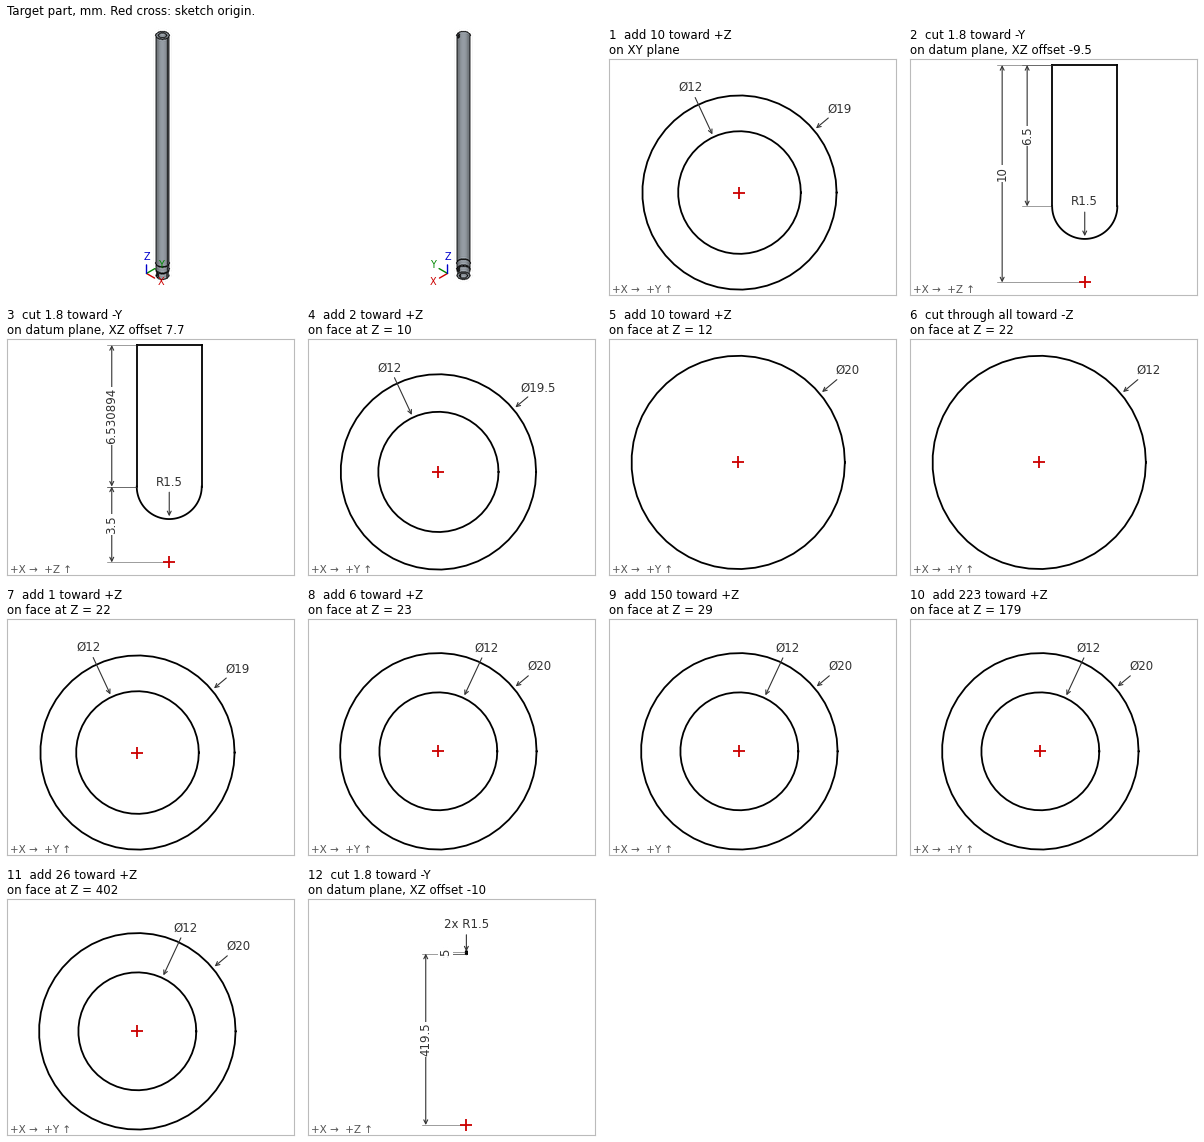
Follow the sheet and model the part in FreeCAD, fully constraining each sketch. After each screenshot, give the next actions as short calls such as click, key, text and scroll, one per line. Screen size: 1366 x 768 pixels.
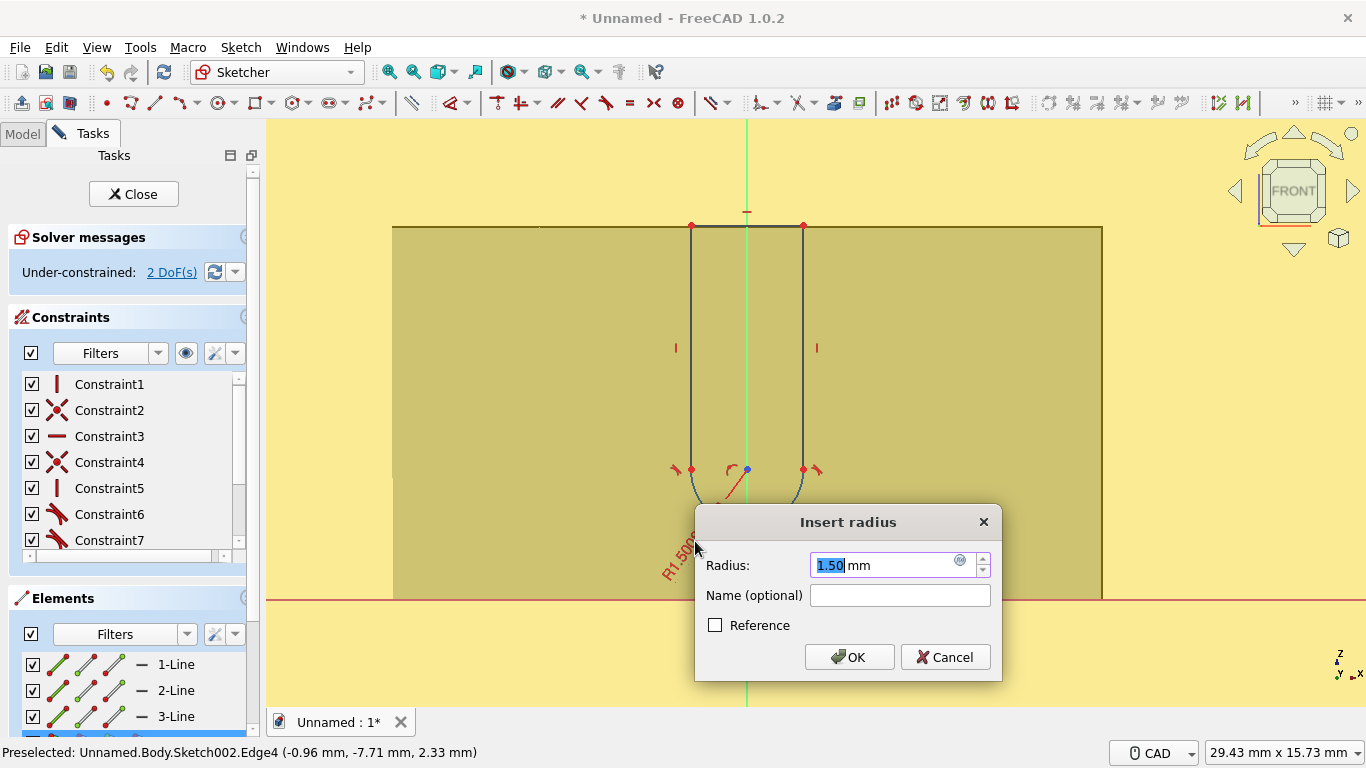
text(1.5)
key(Return)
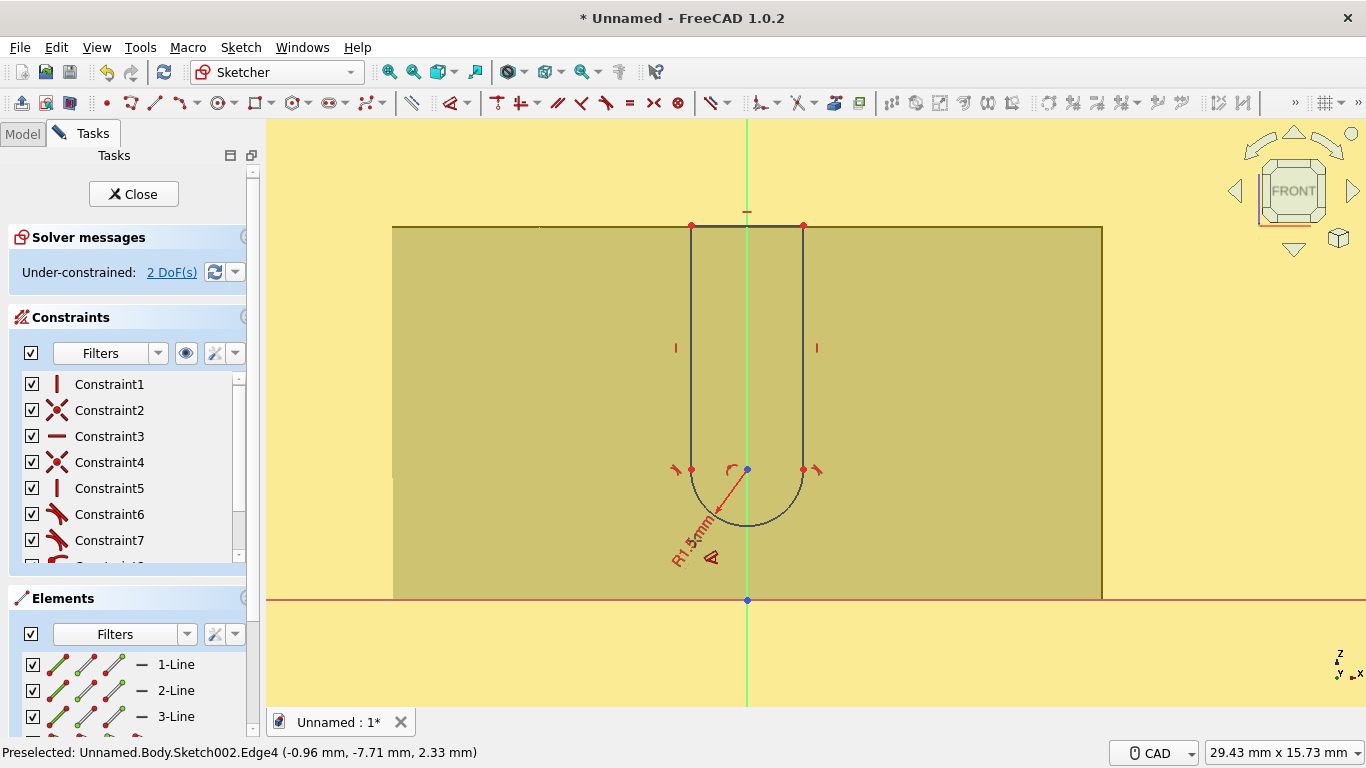
click(691, 470)
click(657, 505)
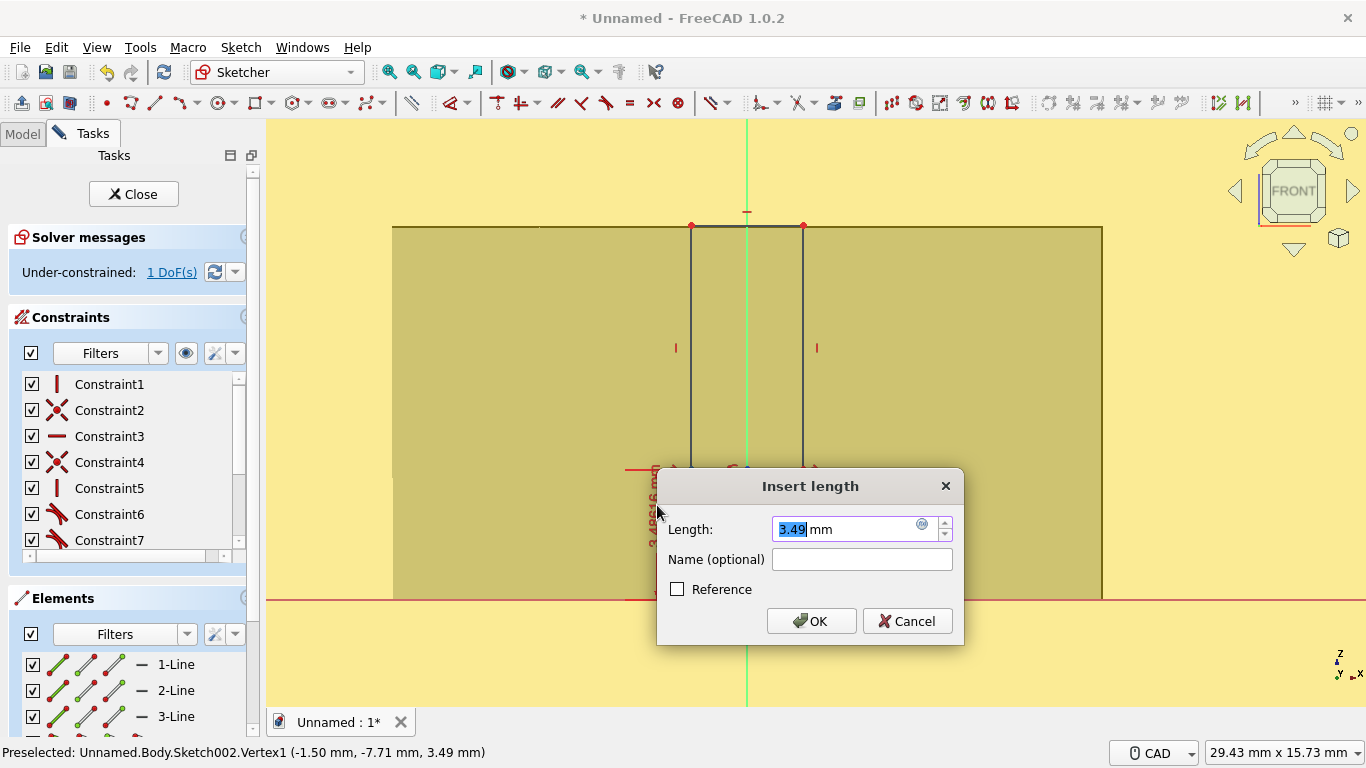
text(3.5)
key(Return)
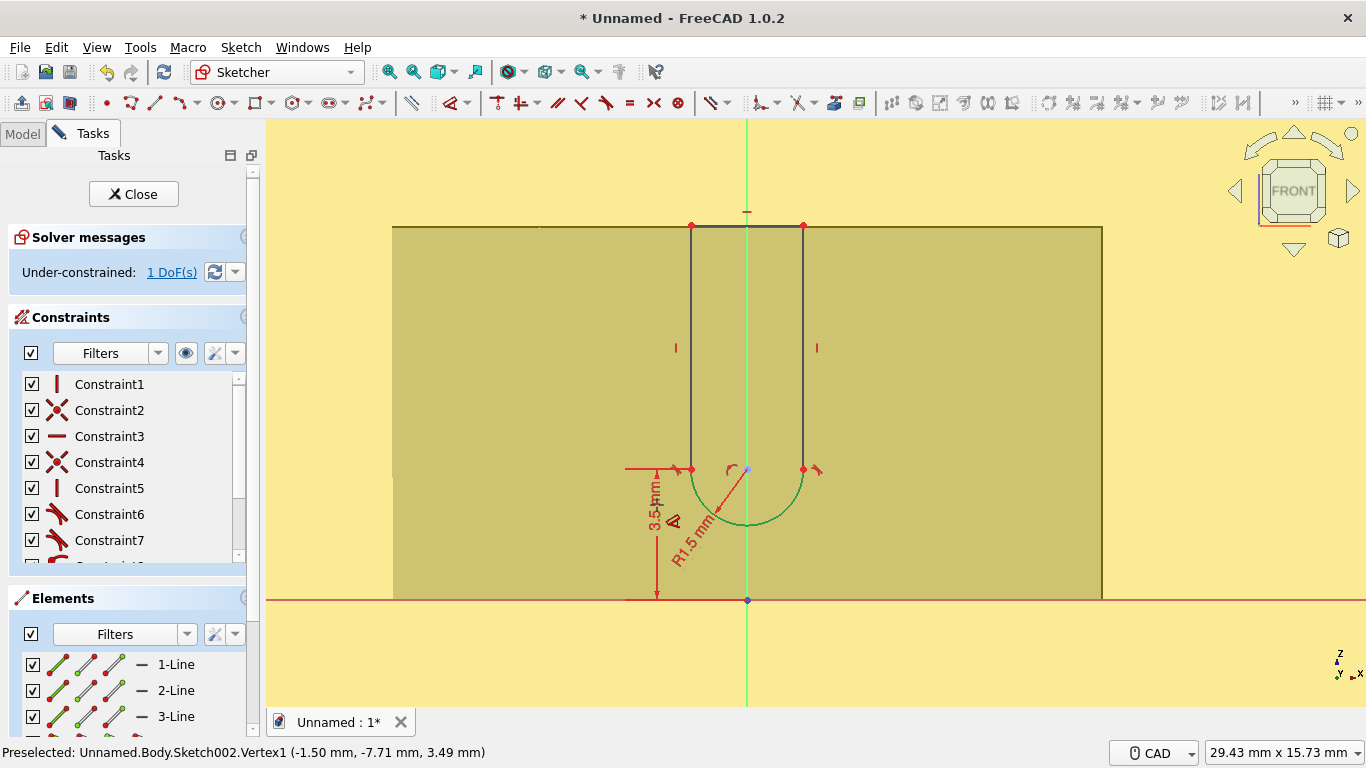
click(691, 396)
click(657, 348)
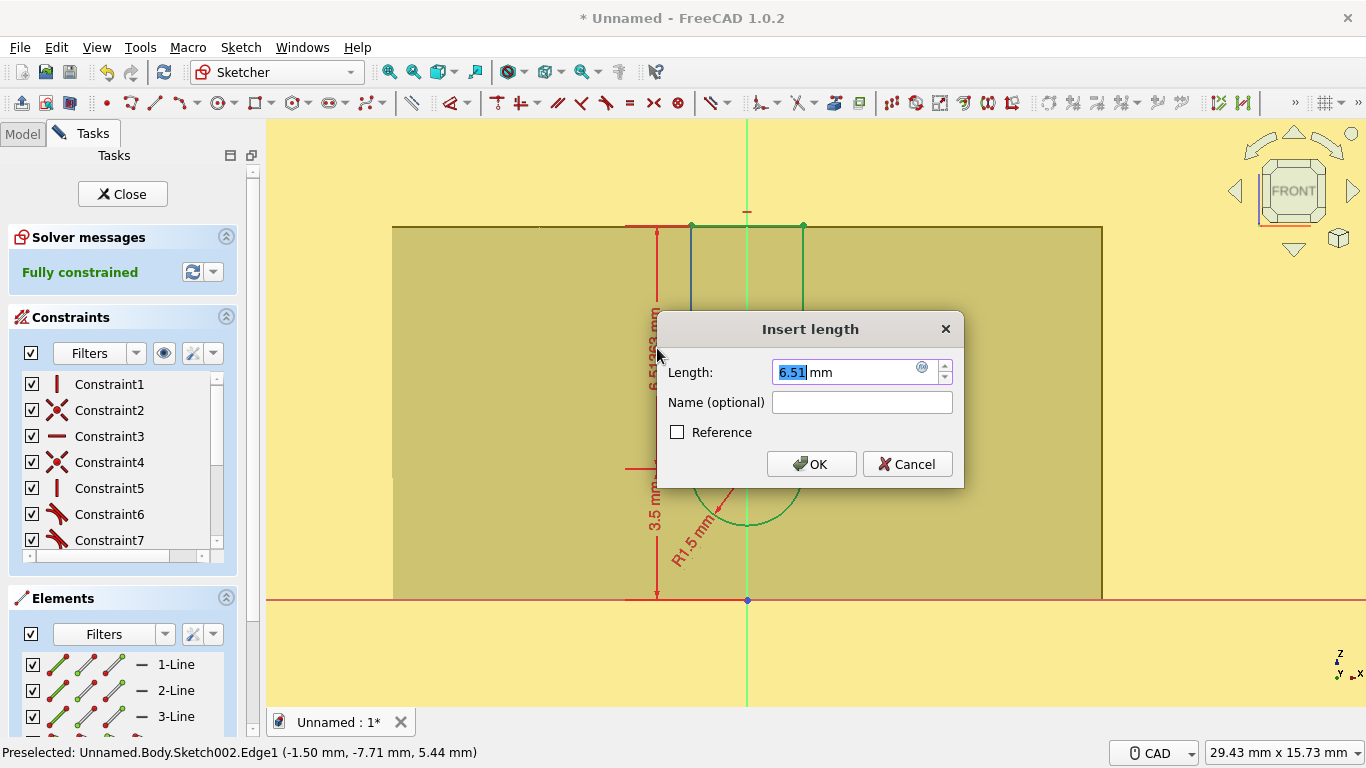
text(6.530894)
key(Return)
key(Escape)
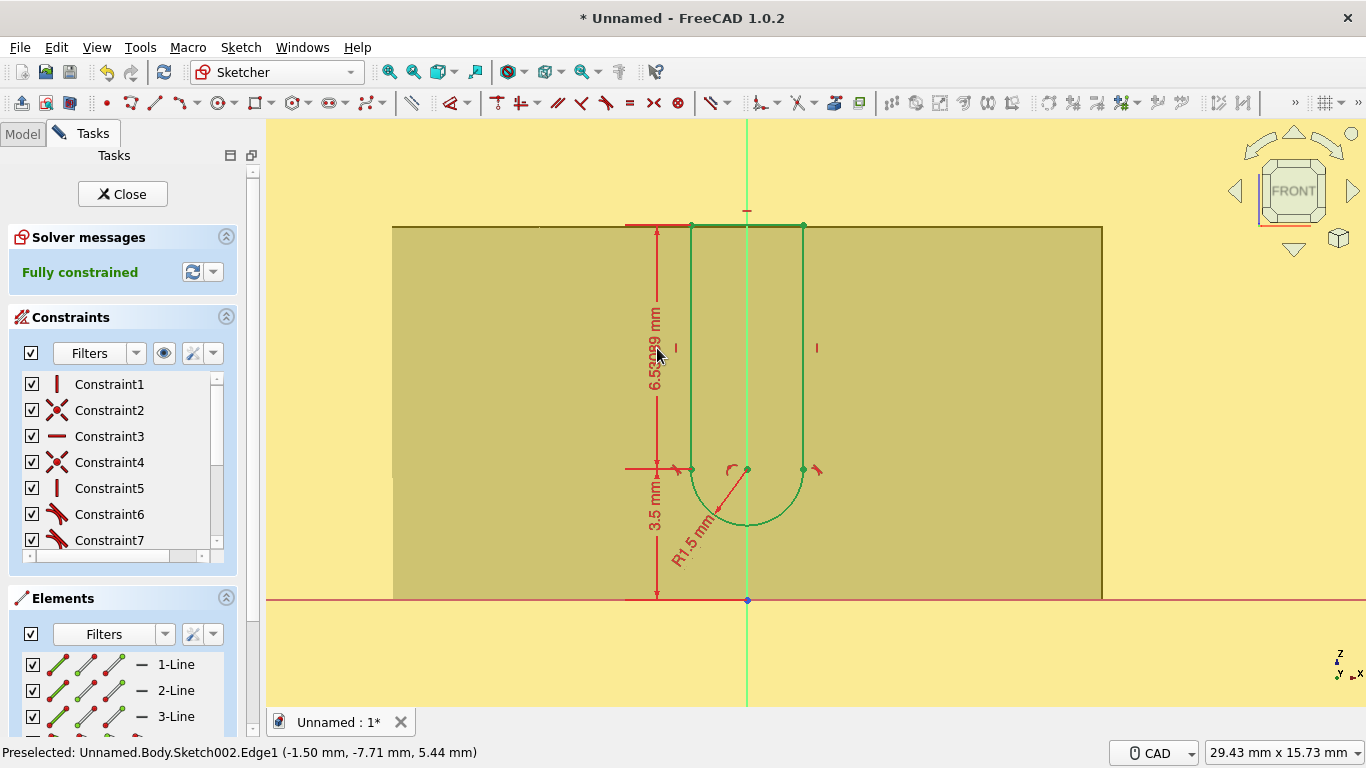
click(123, 194)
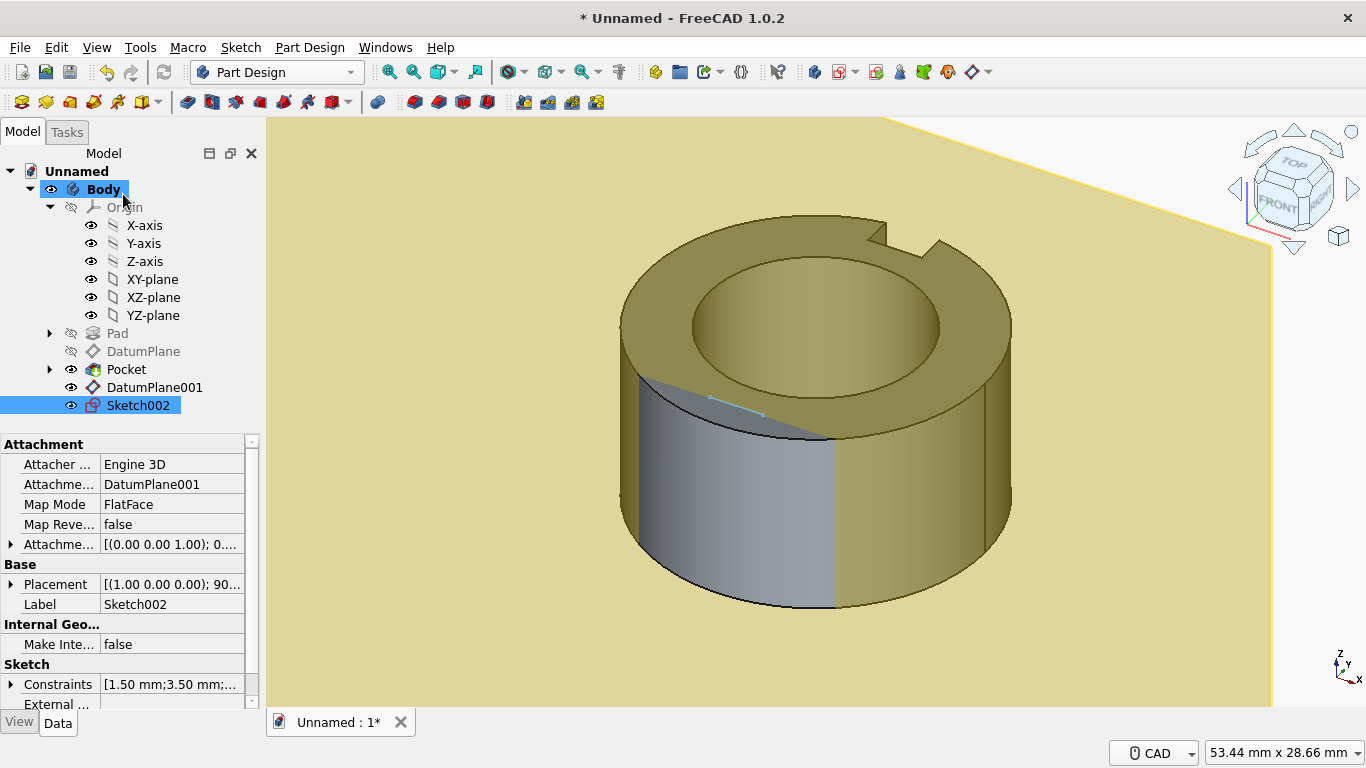
click(188, 102)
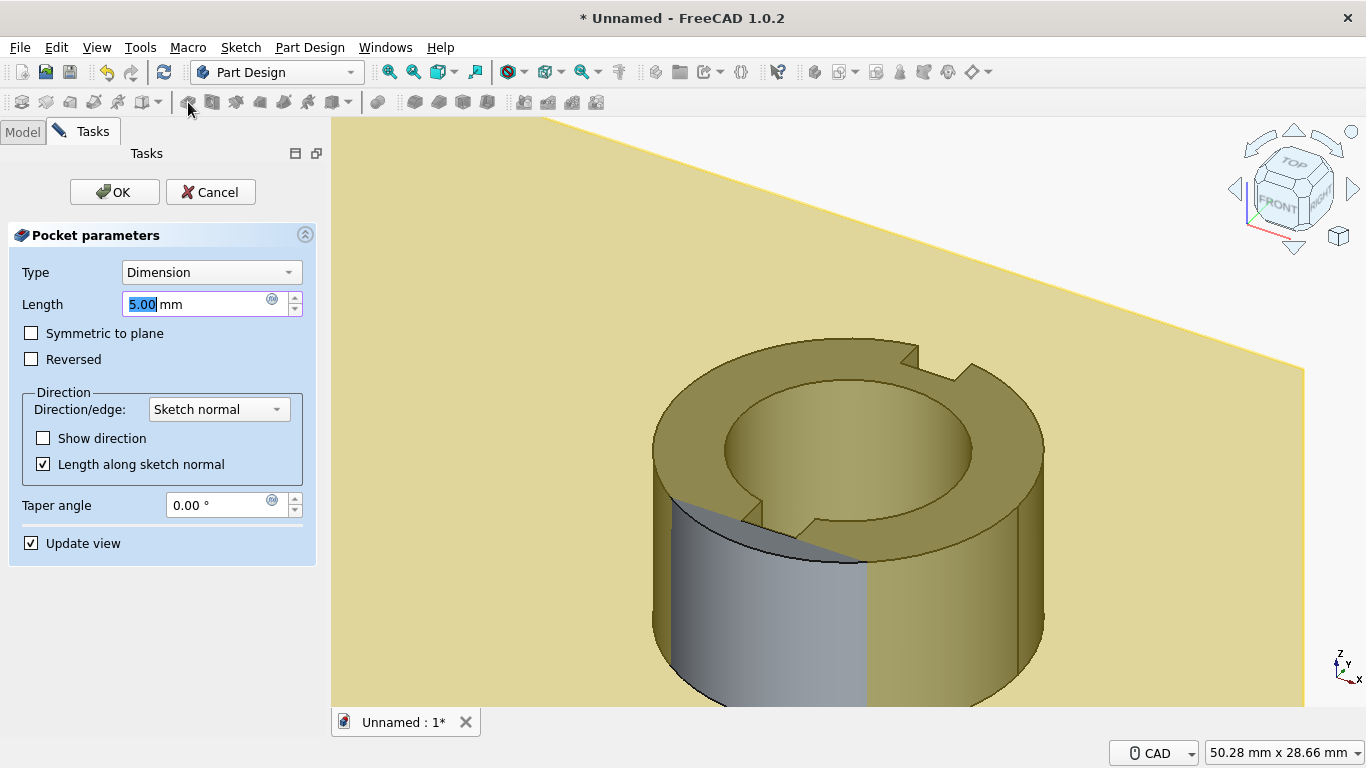
text(1.8)
key(Tab)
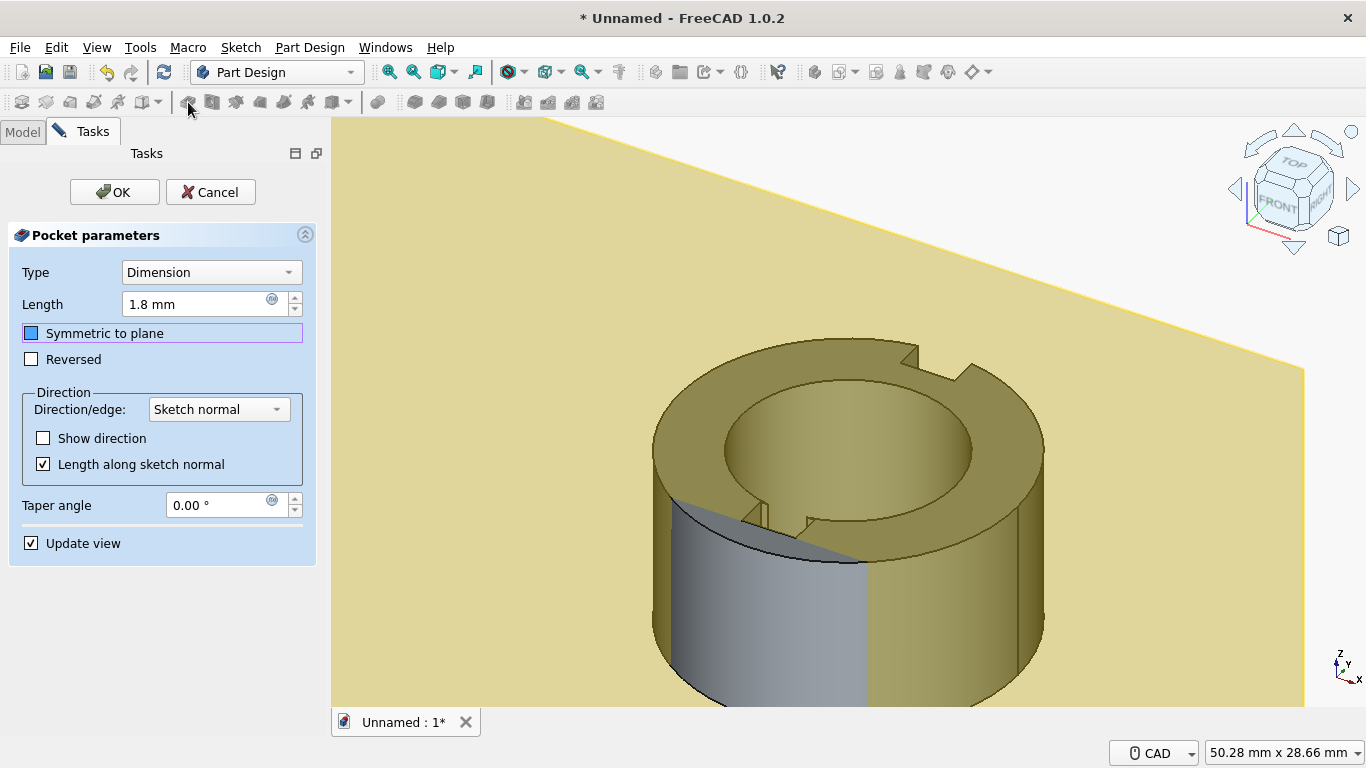
click(30, 359)